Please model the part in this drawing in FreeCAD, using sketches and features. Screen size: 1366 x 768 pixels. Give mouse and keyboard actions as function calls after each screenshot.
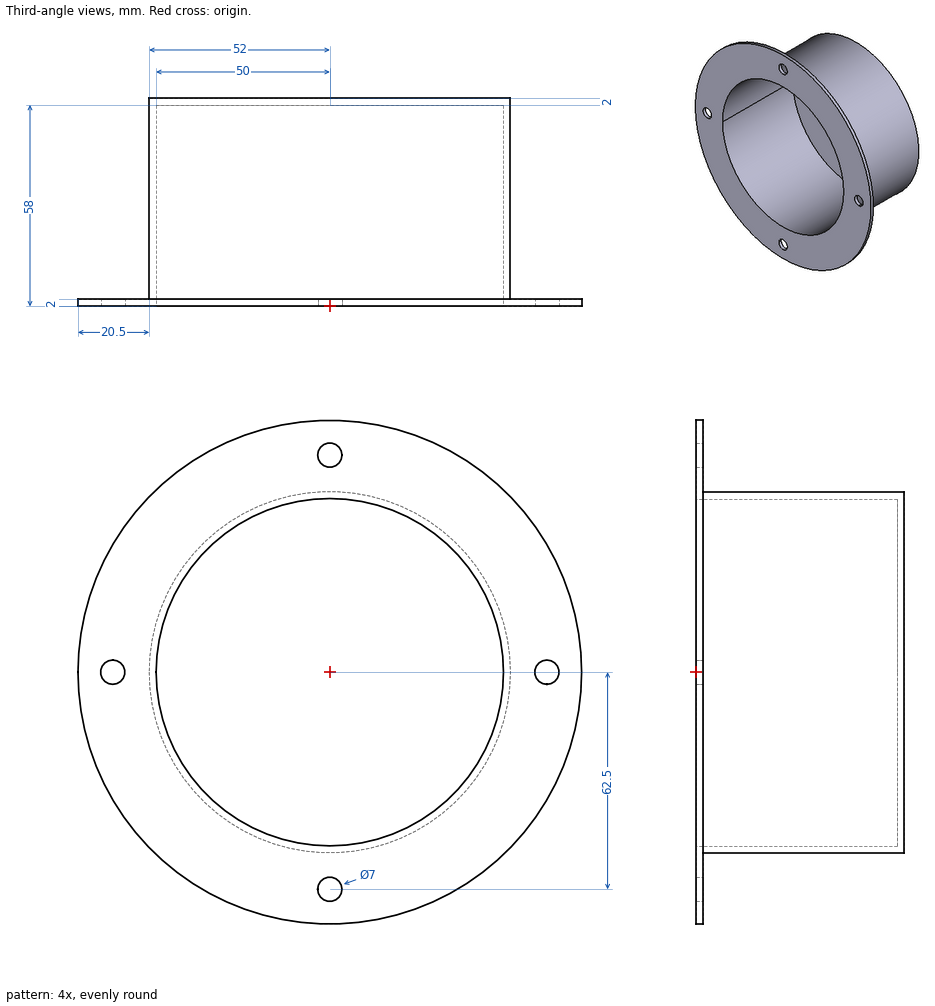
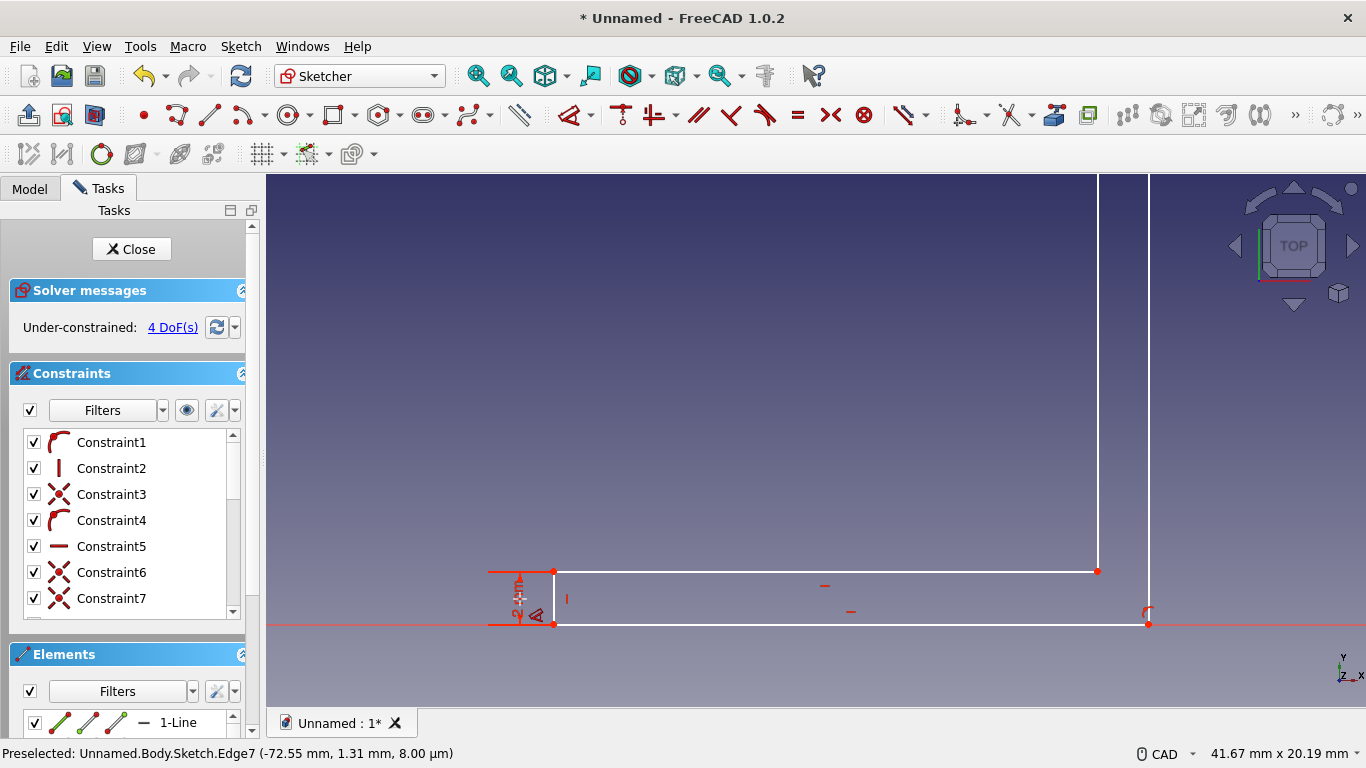
scroll(554, 594, down, 8)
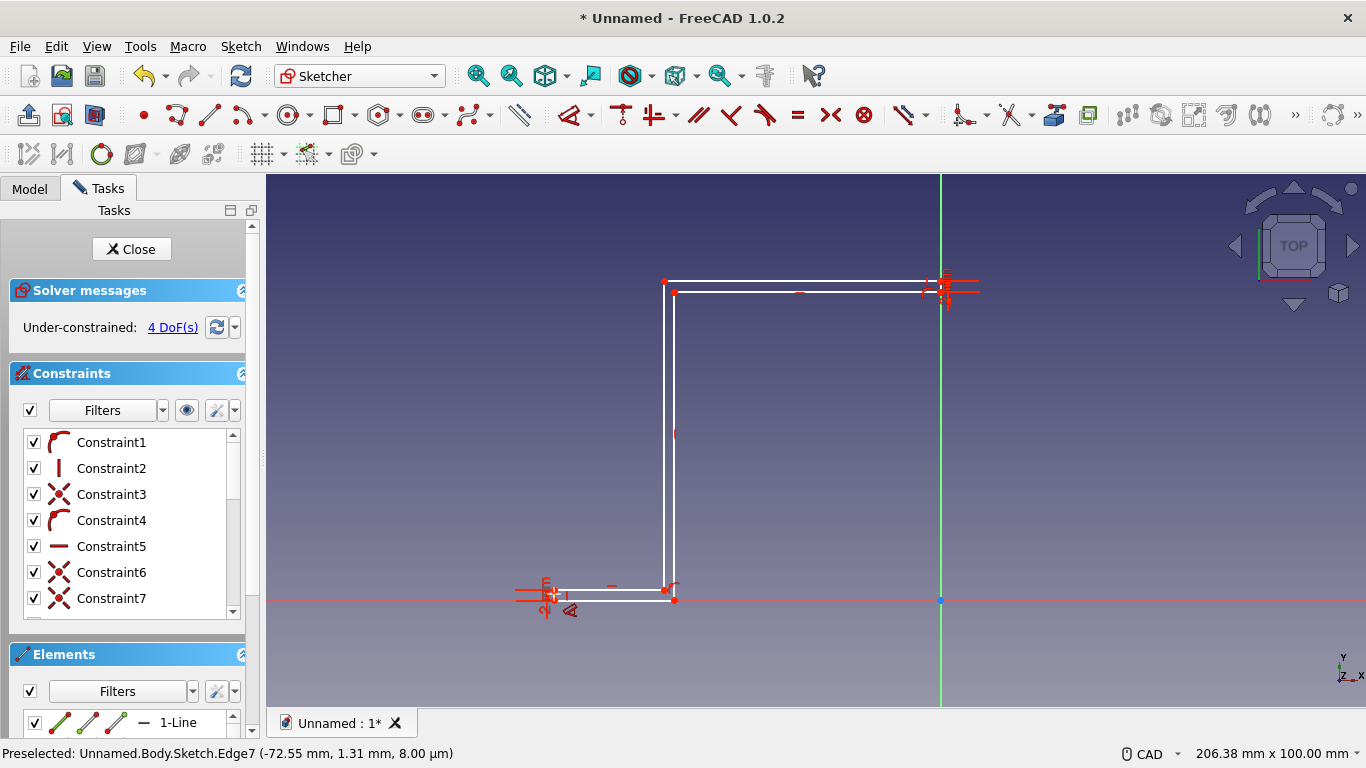
scroll(674, 539, up, 2)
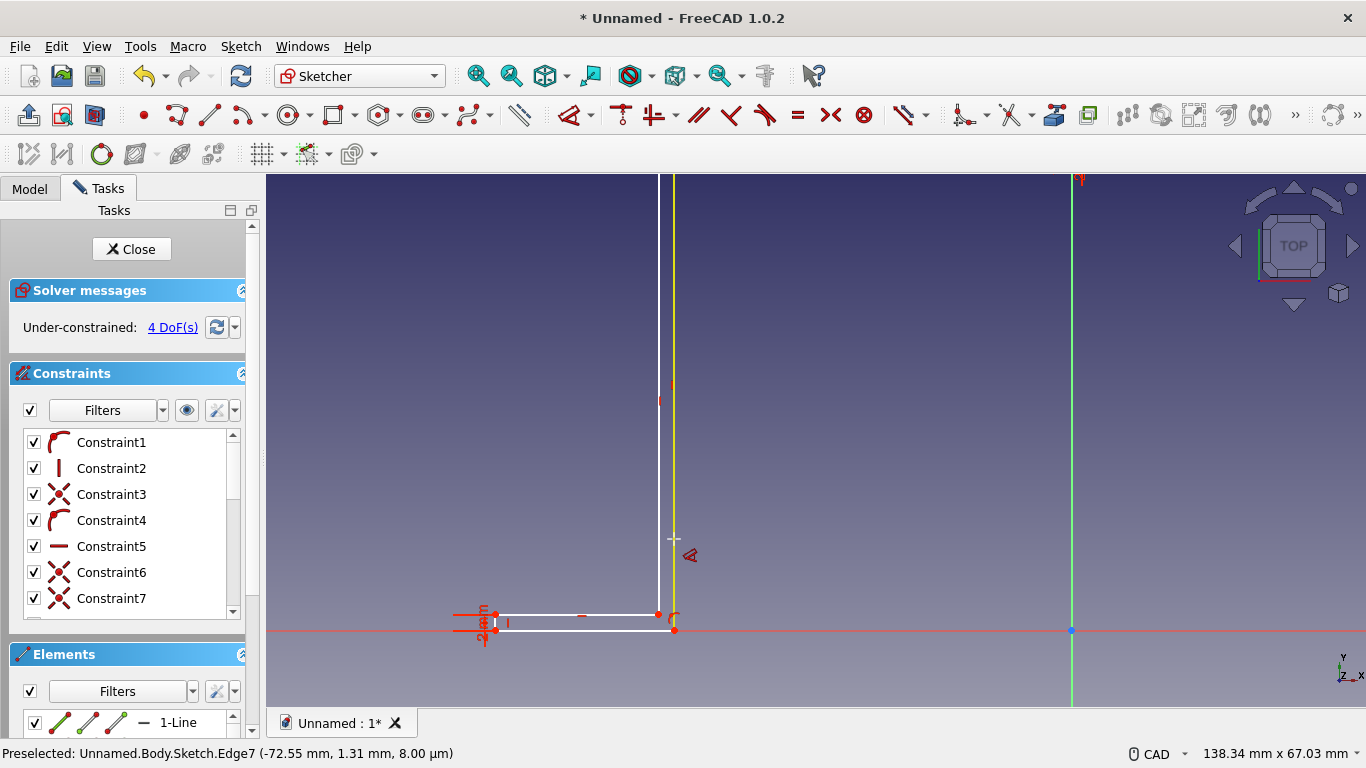
click(674, 539)
click(640, 416)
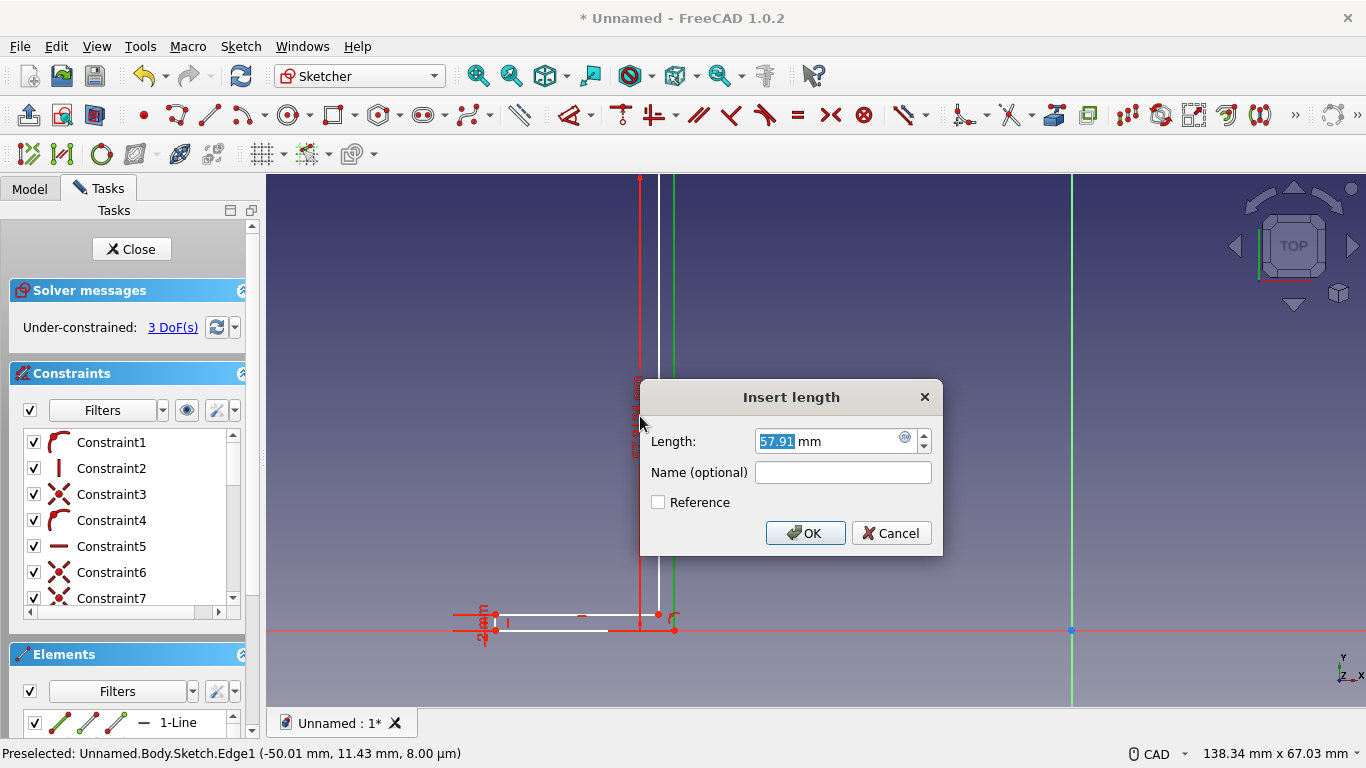
text(58)
key(Return)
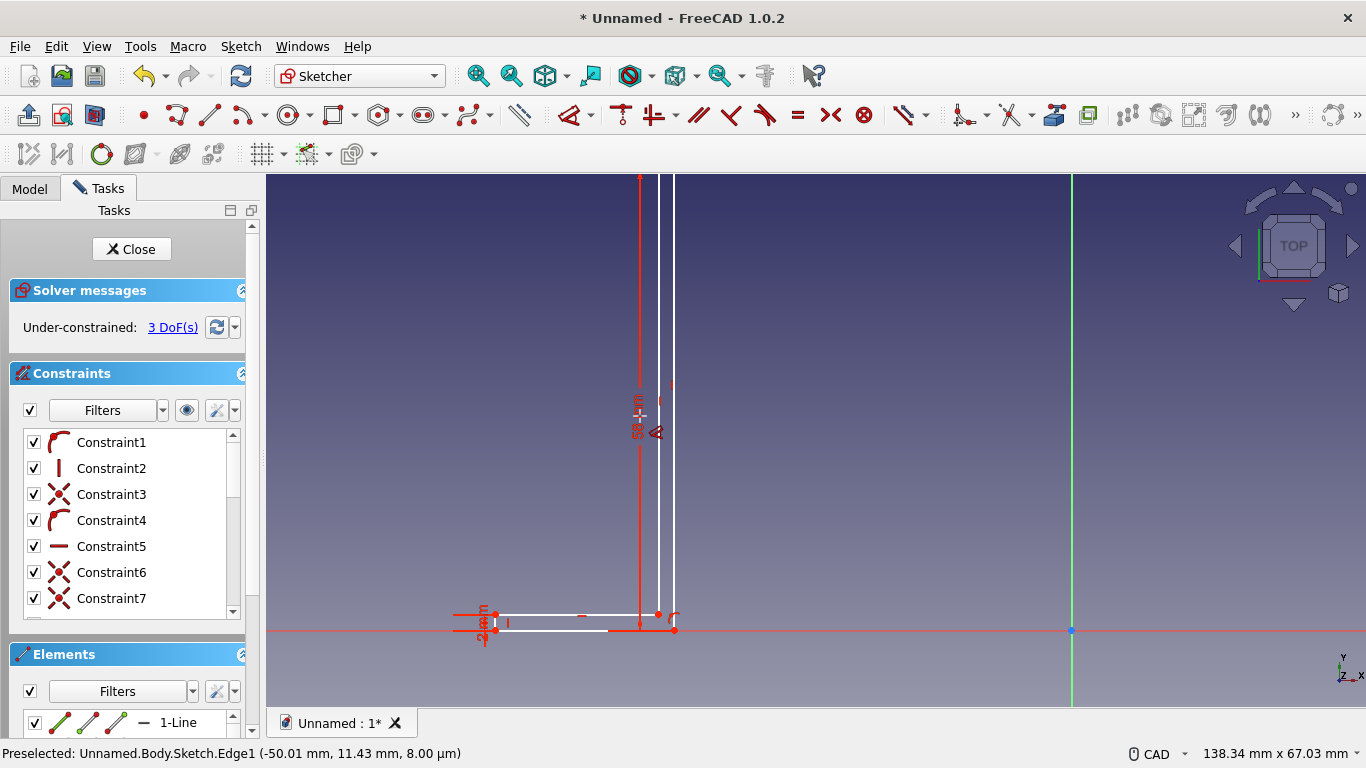
scroll(674, 538, down, 2)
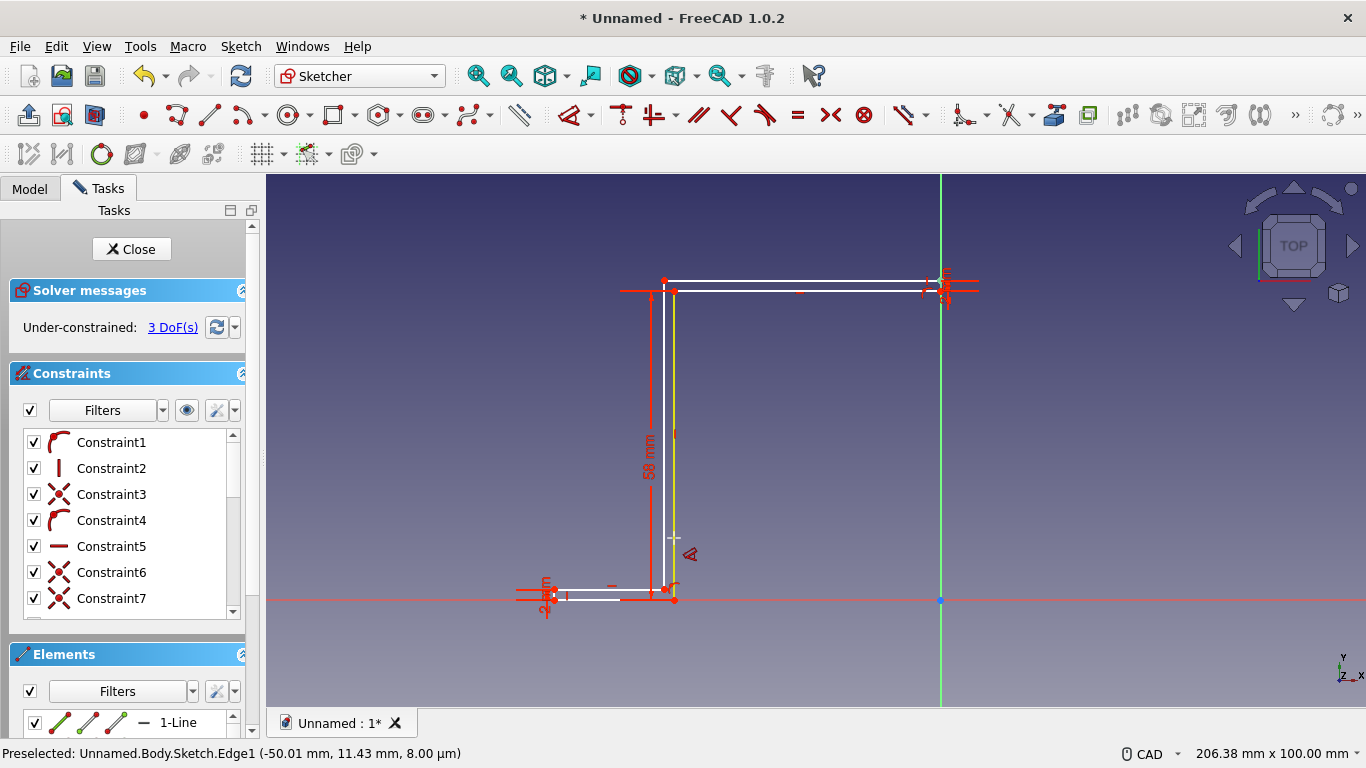
scroll(754, 291, up, 2)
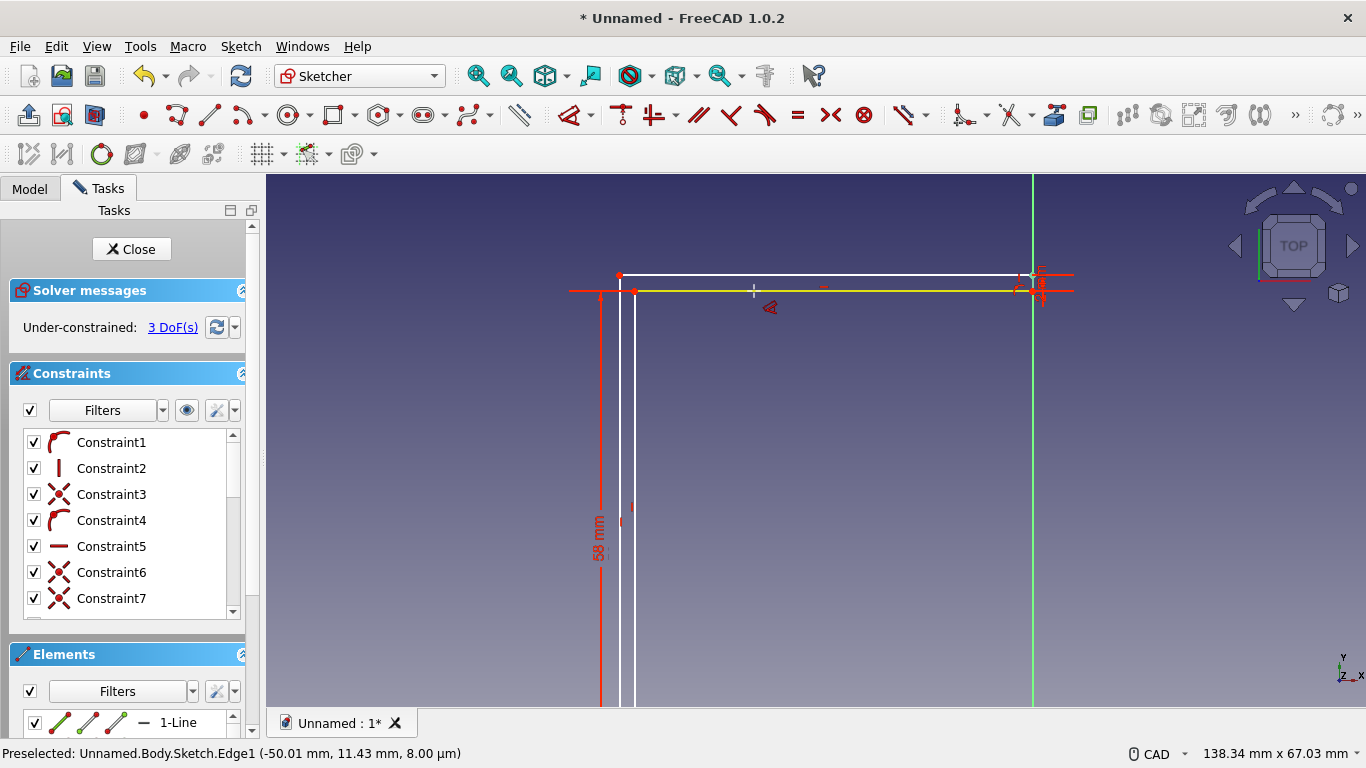
click(754, 291)
click(834, 257)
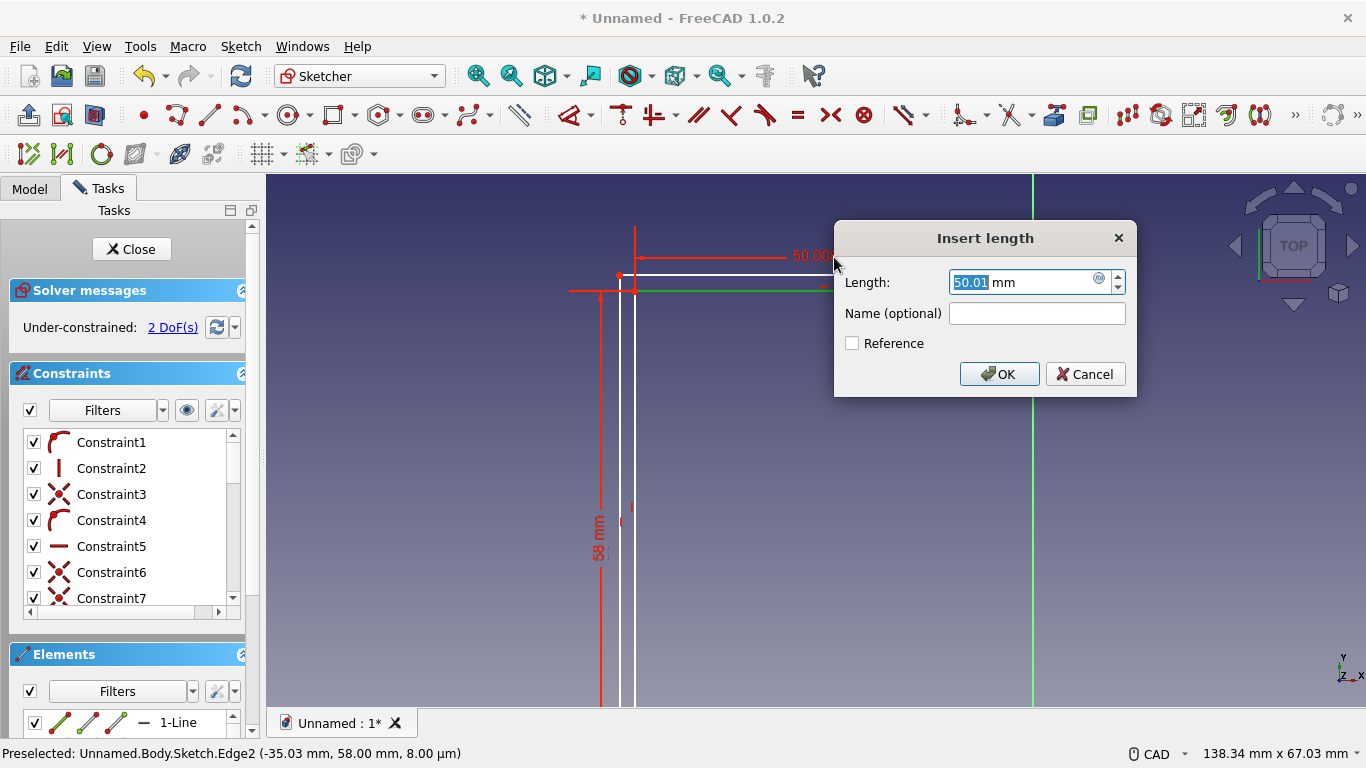
text(50)
key(Return)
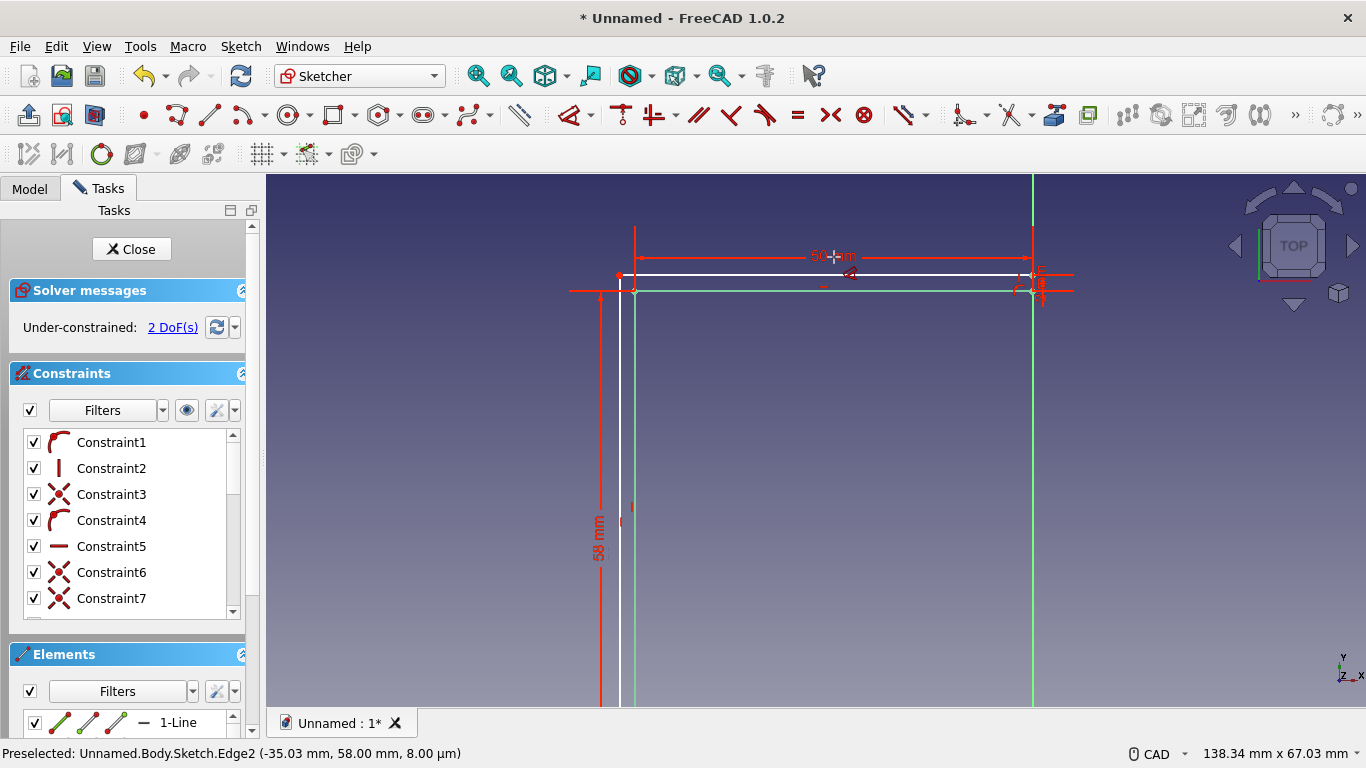
click(909, 275)
click(731, 241)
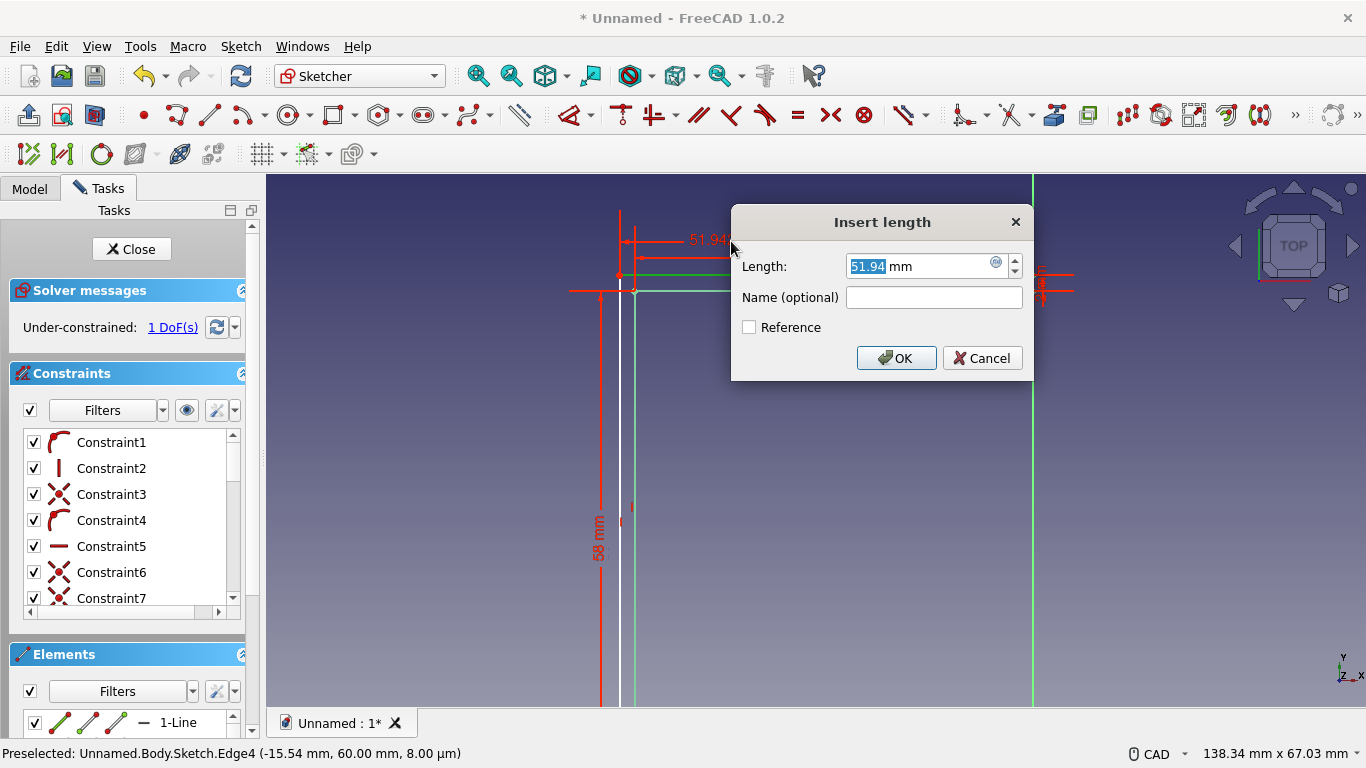
text(52)
key(Return)